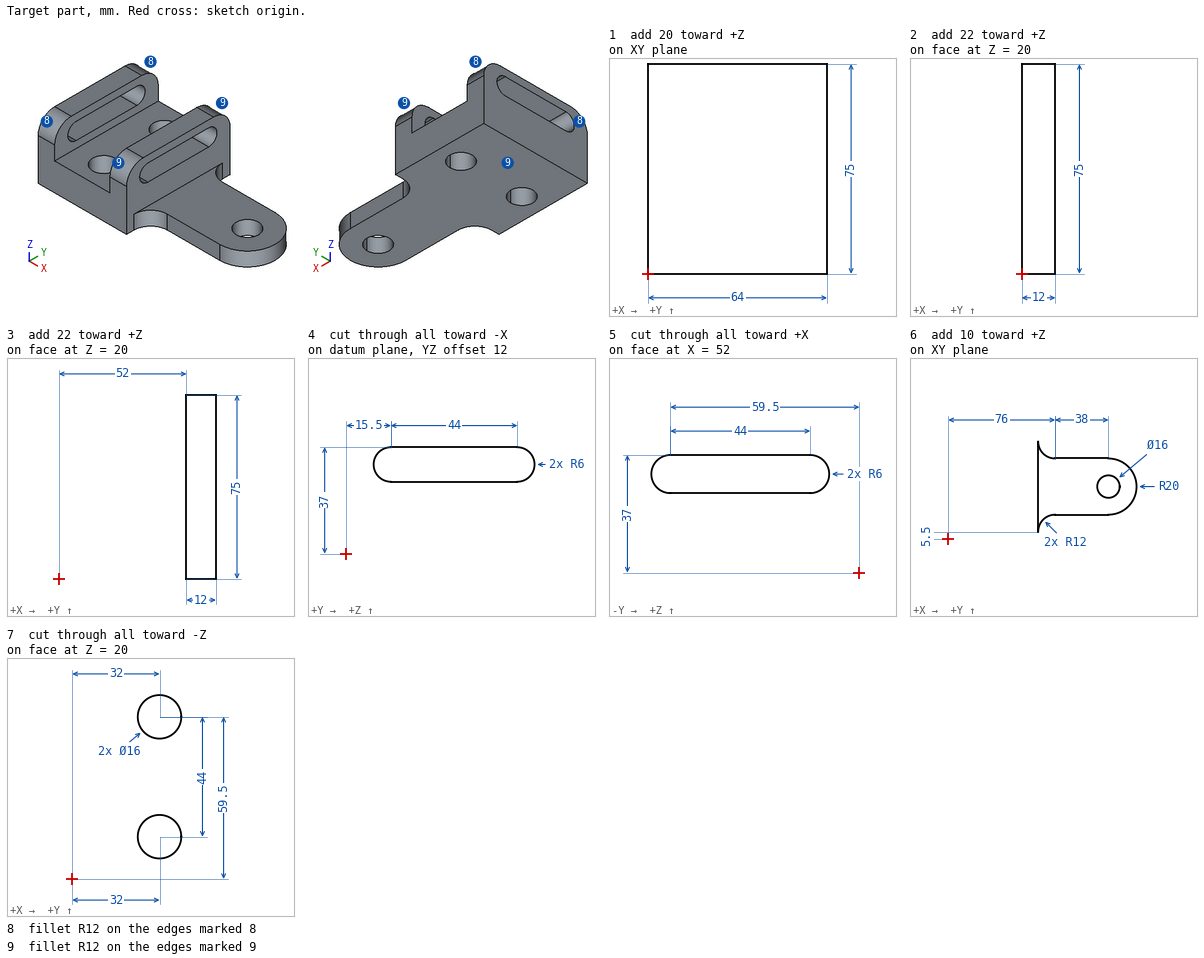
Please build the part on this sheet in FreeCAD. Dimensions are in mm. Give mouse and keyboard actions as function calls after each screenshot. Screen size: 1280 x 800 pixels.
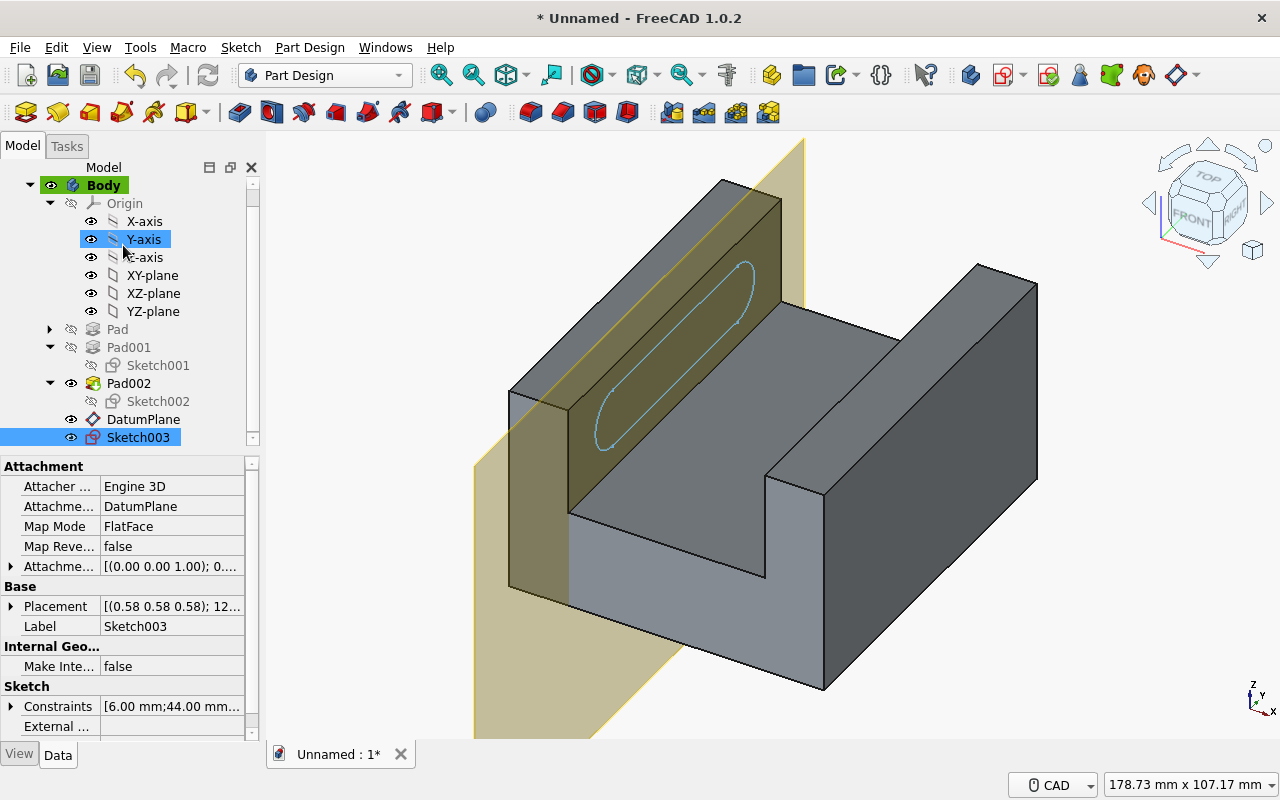
click(240, 112)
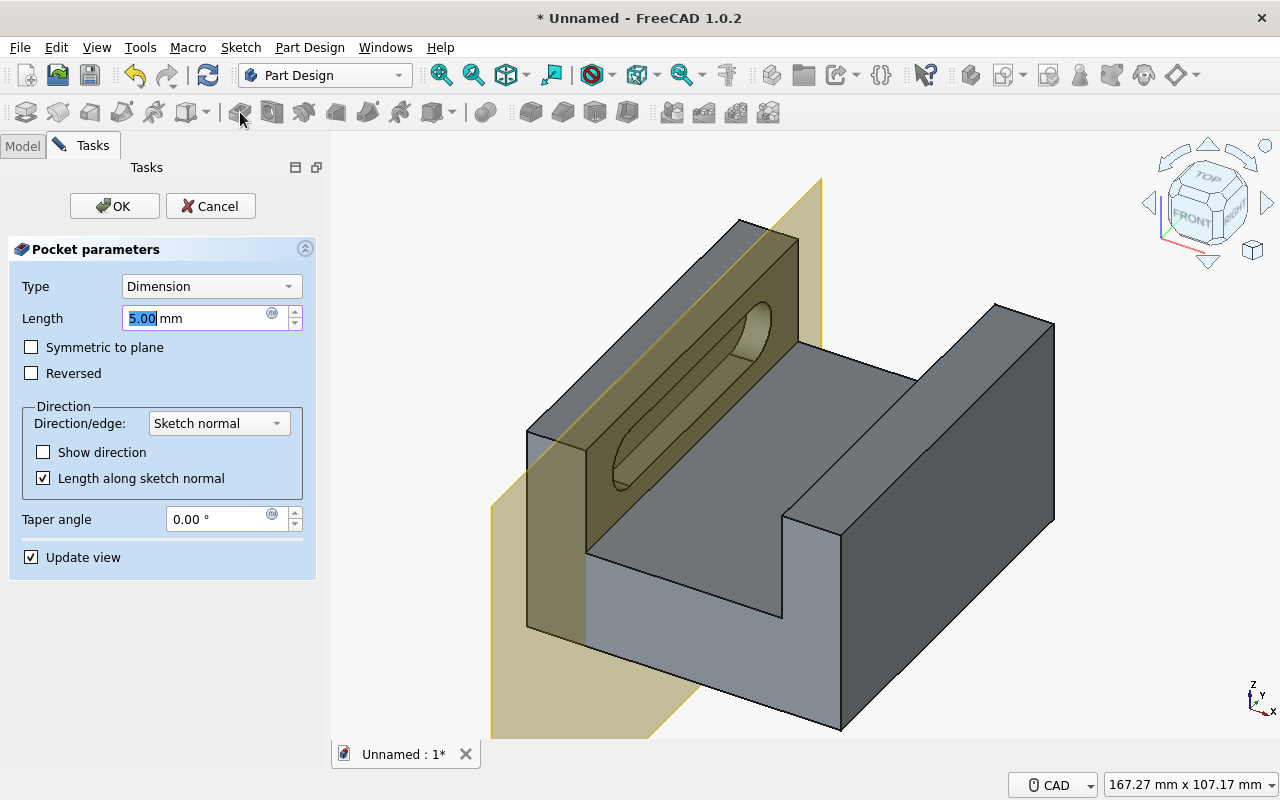
click(212, 286)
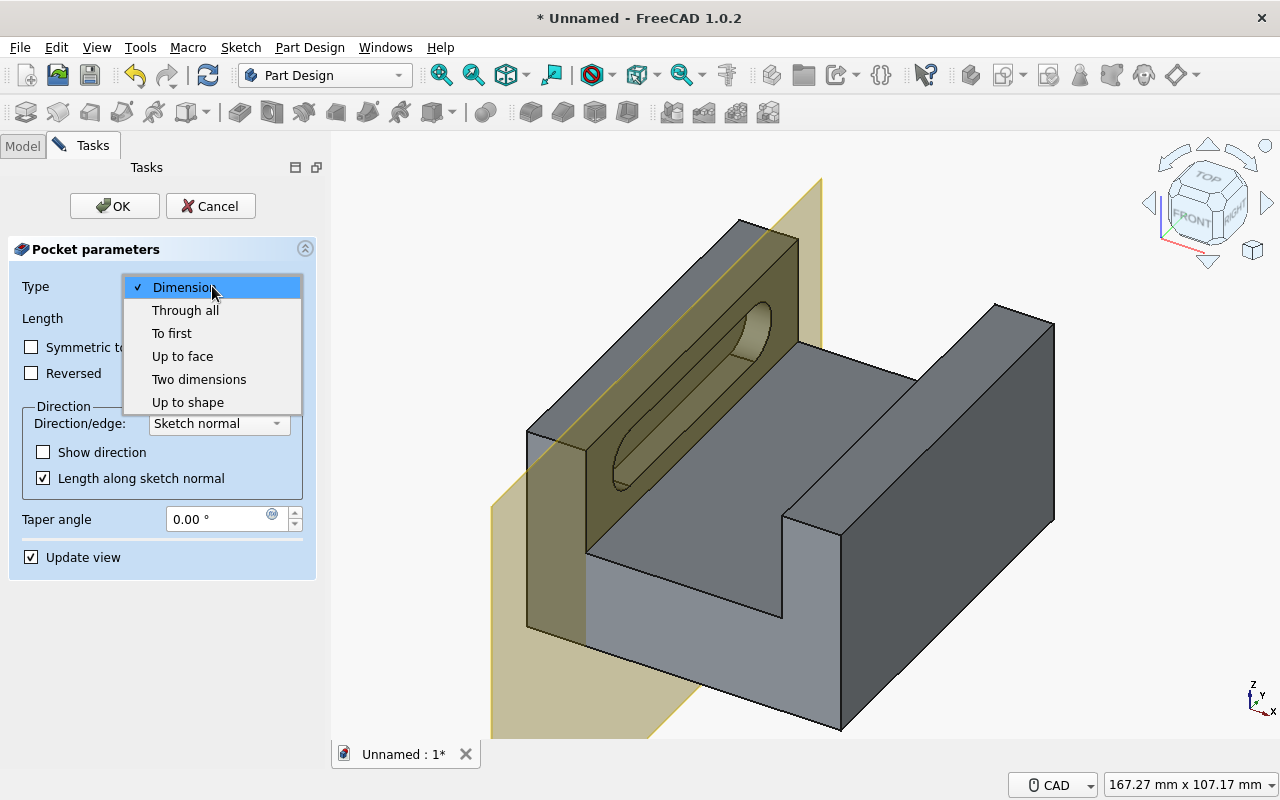
click(212, 310)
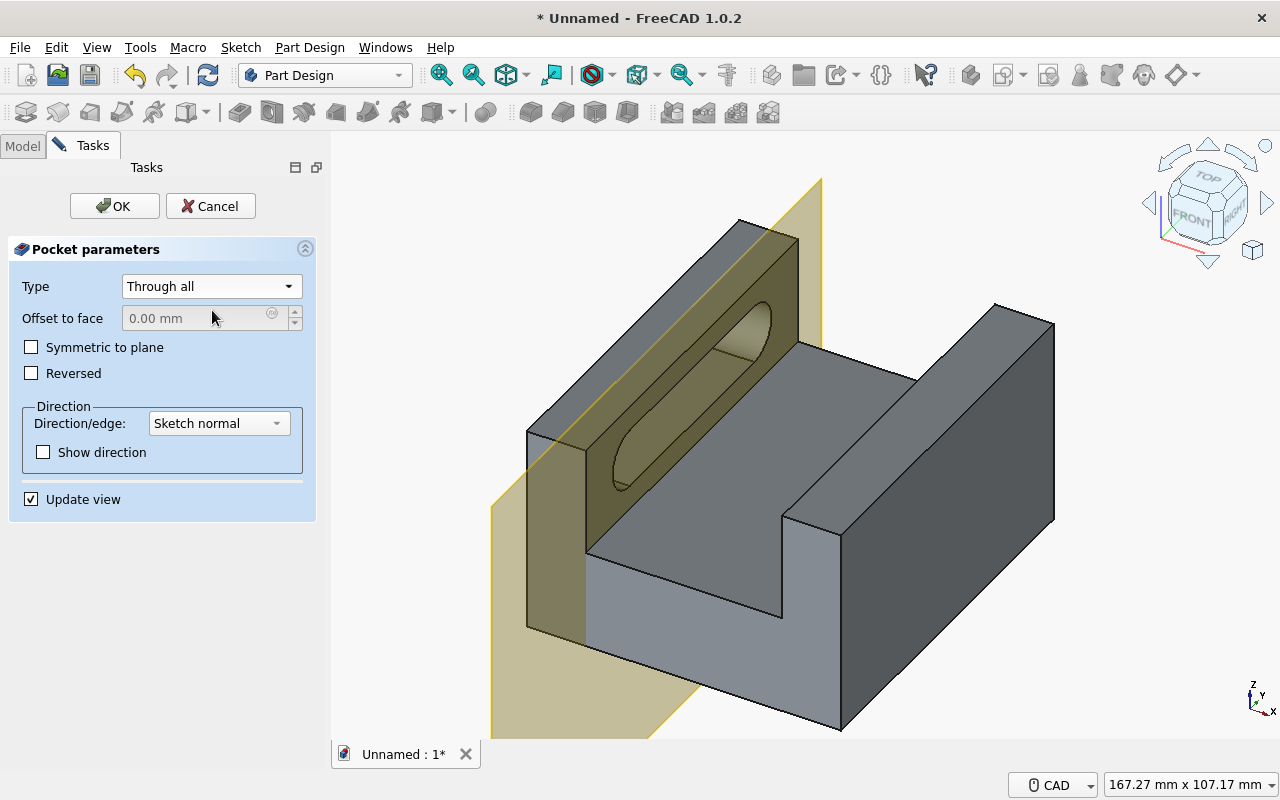
click(115, 206)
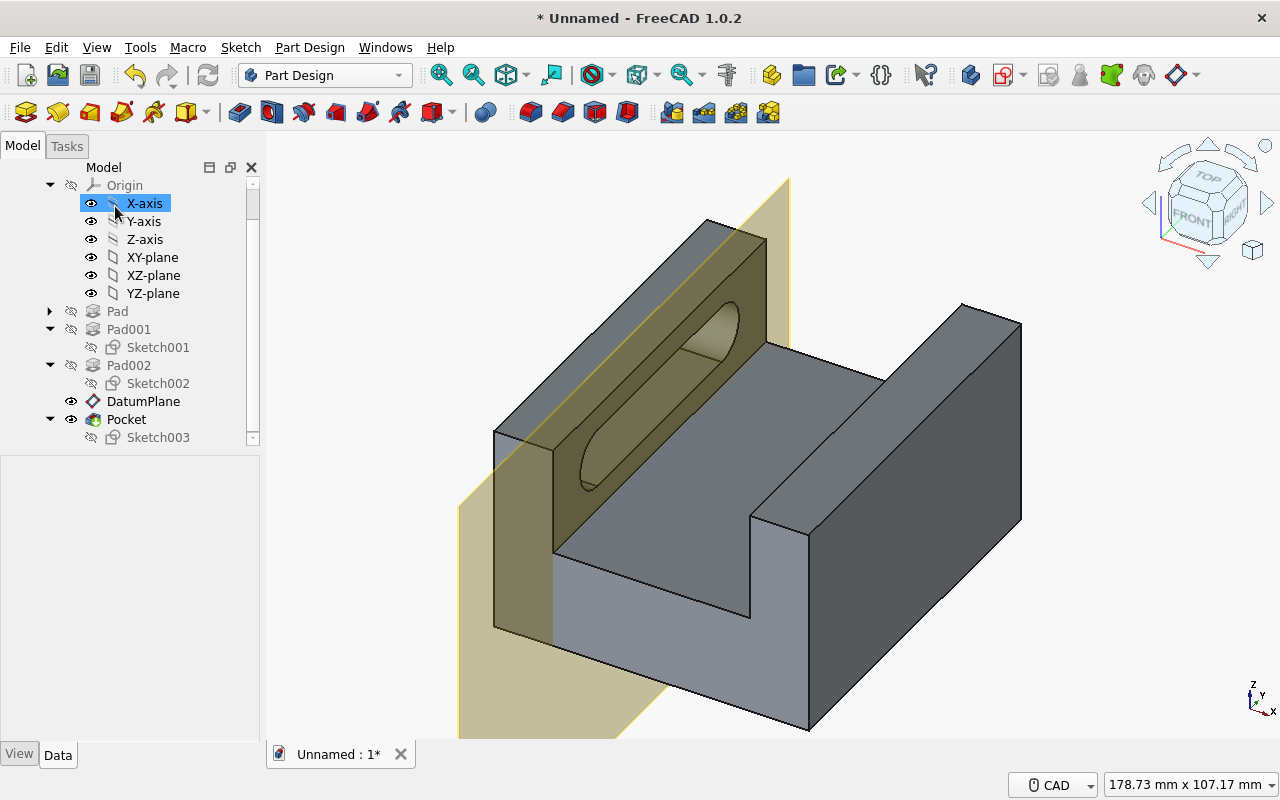
click(116, 401)
key(space)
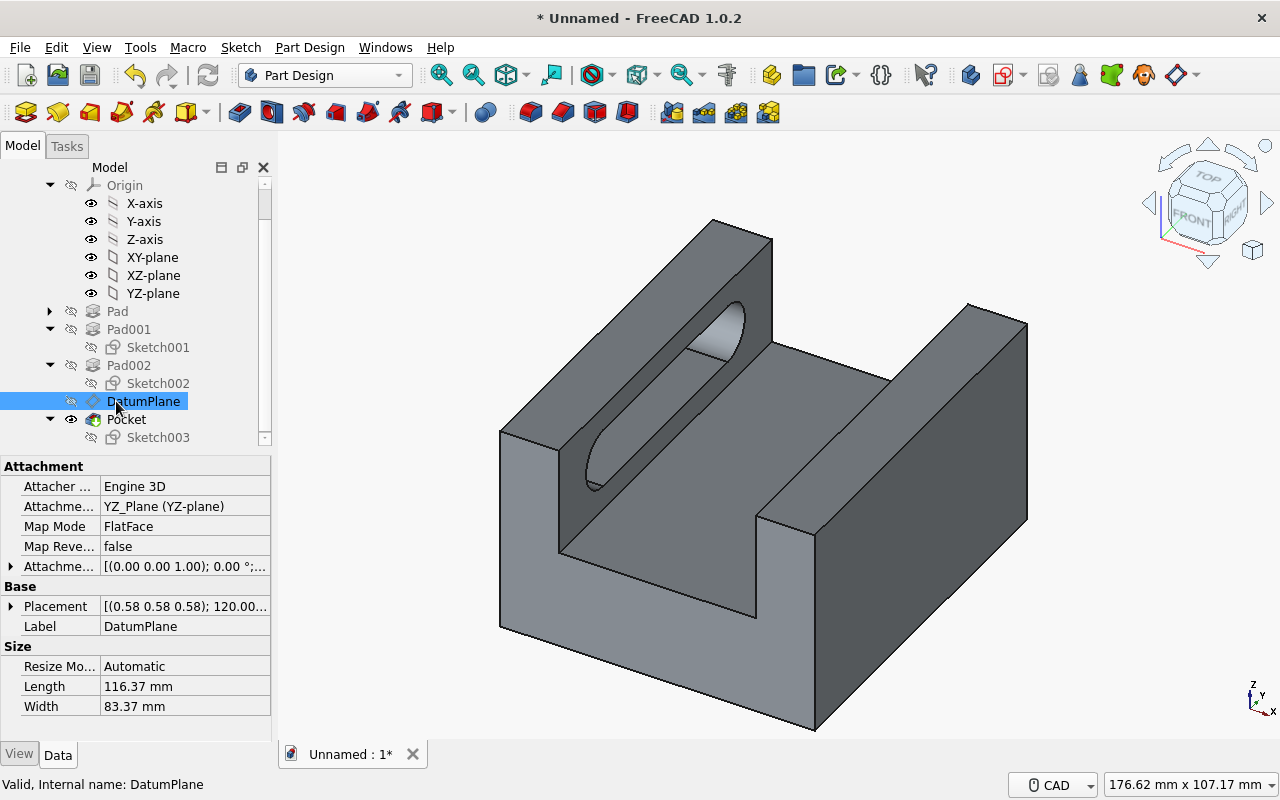
key(6)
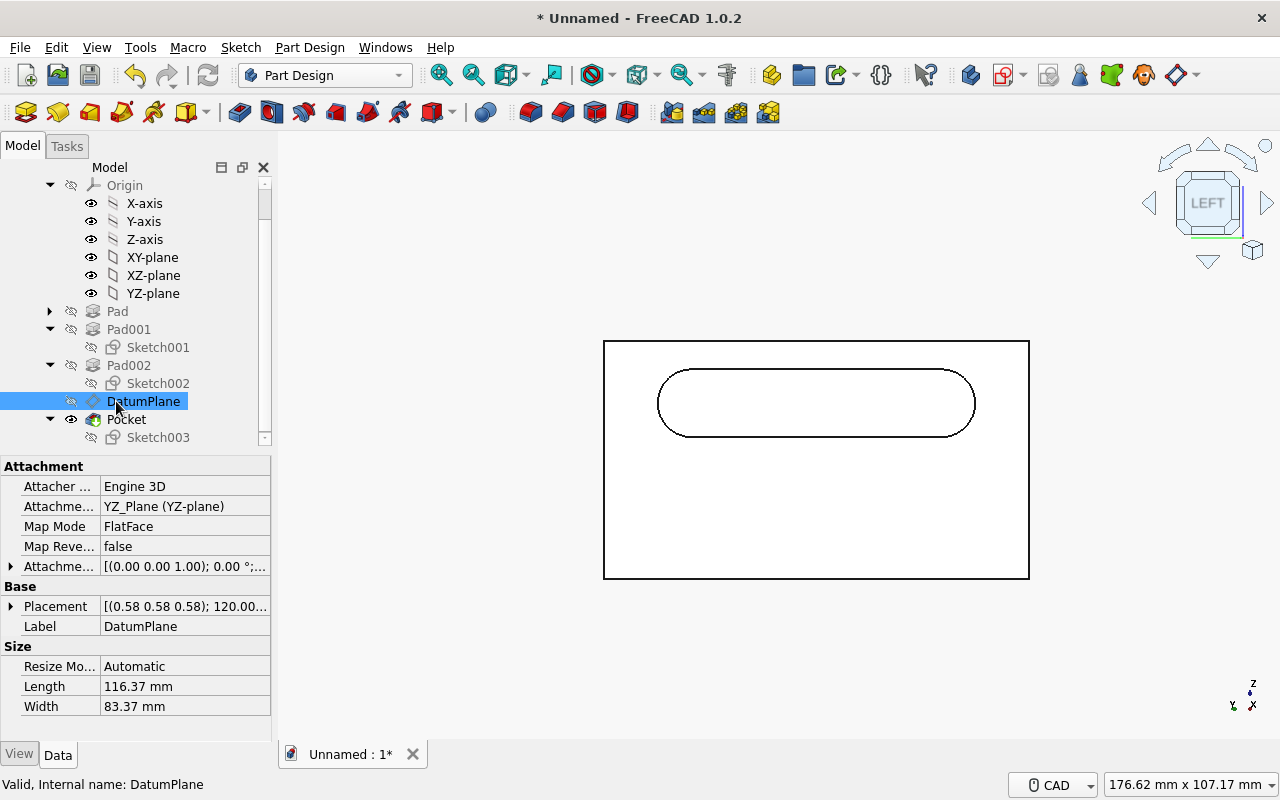
click(442, 76)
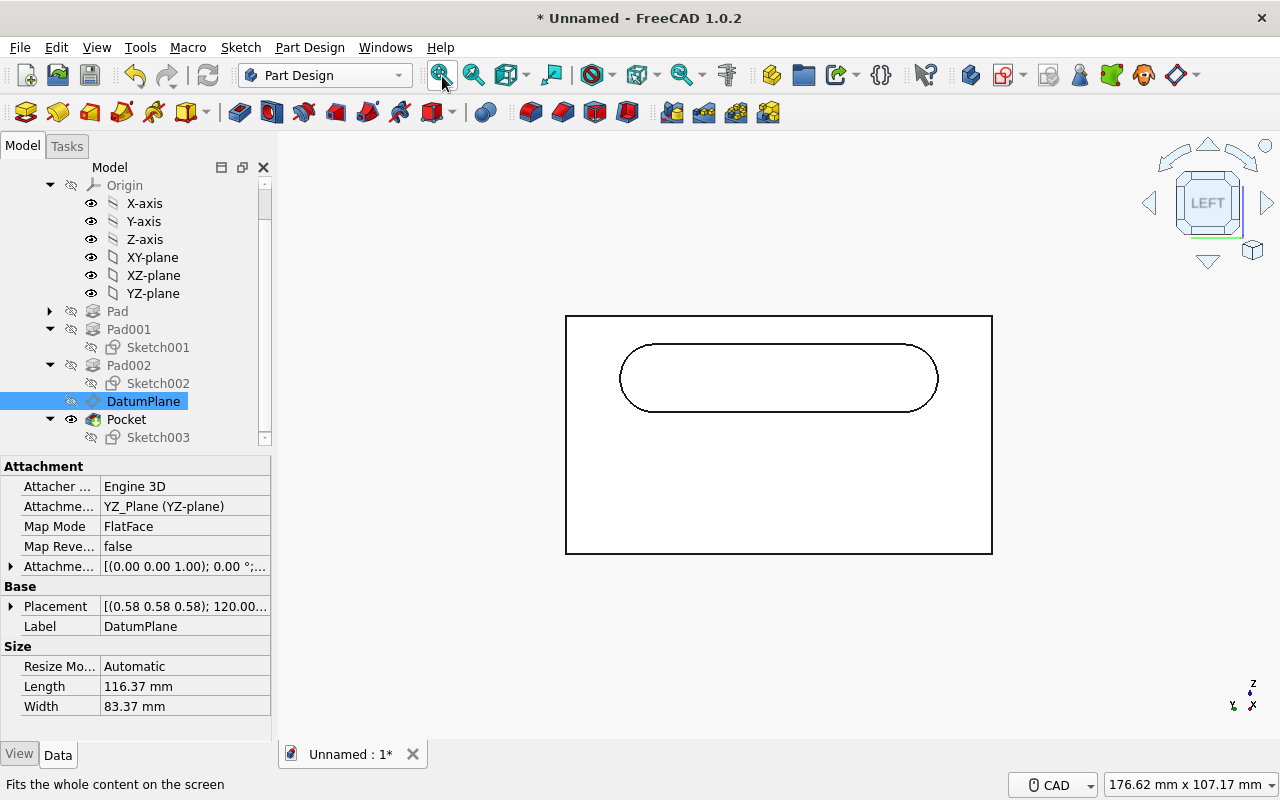
click(657, 377)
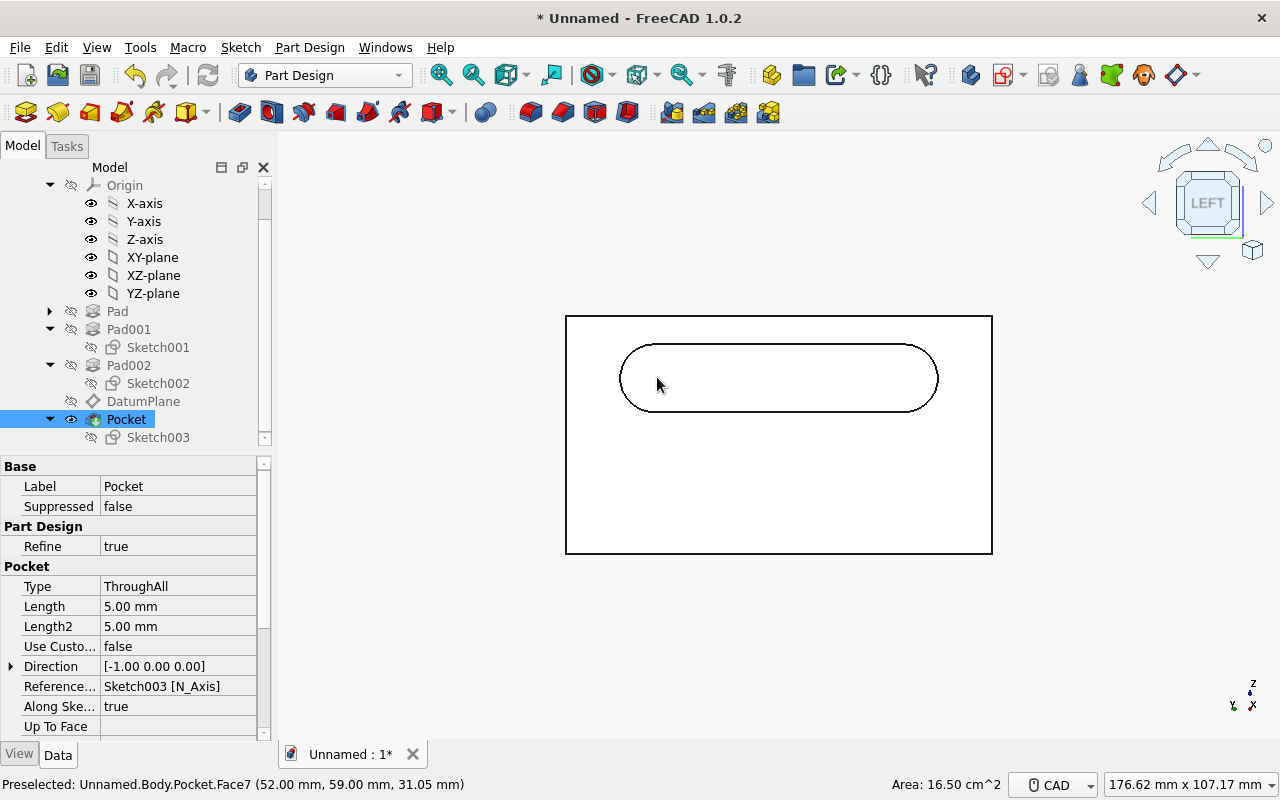
click(1004, 76)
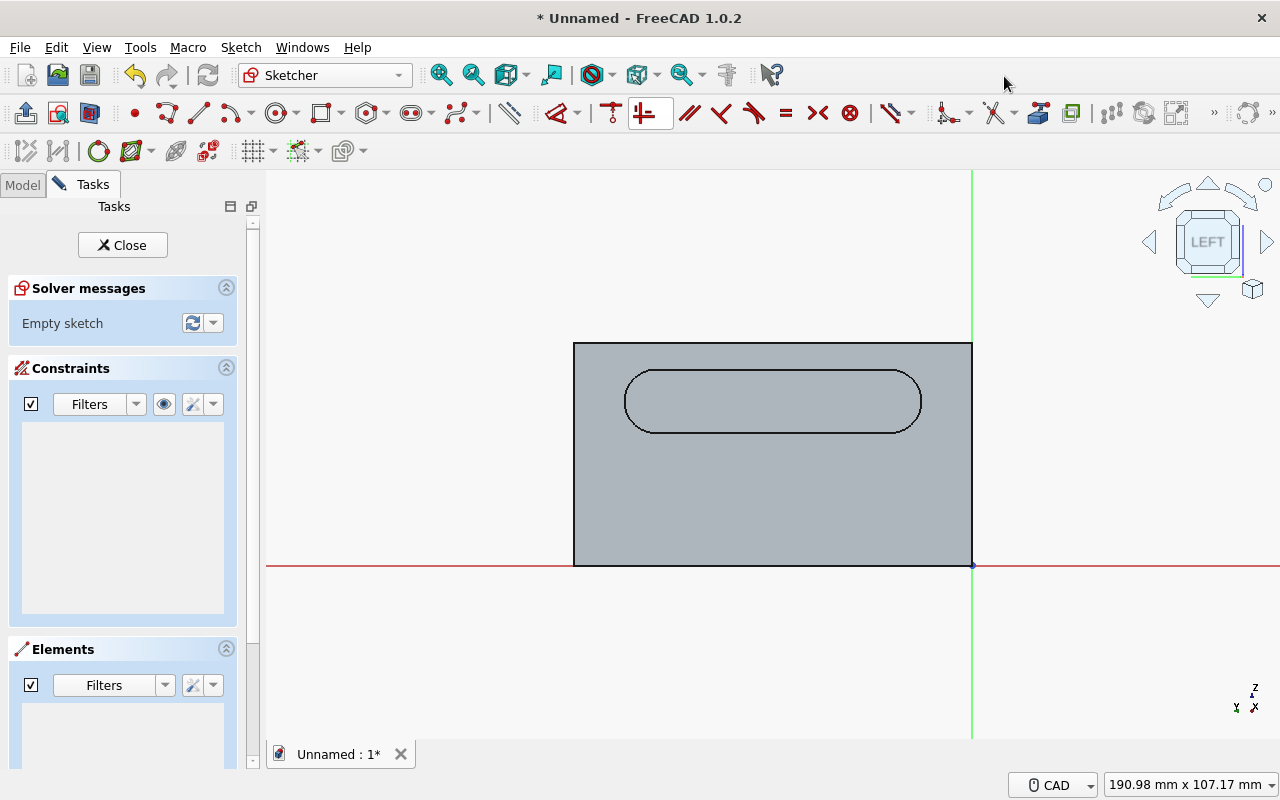
click(90, 114)